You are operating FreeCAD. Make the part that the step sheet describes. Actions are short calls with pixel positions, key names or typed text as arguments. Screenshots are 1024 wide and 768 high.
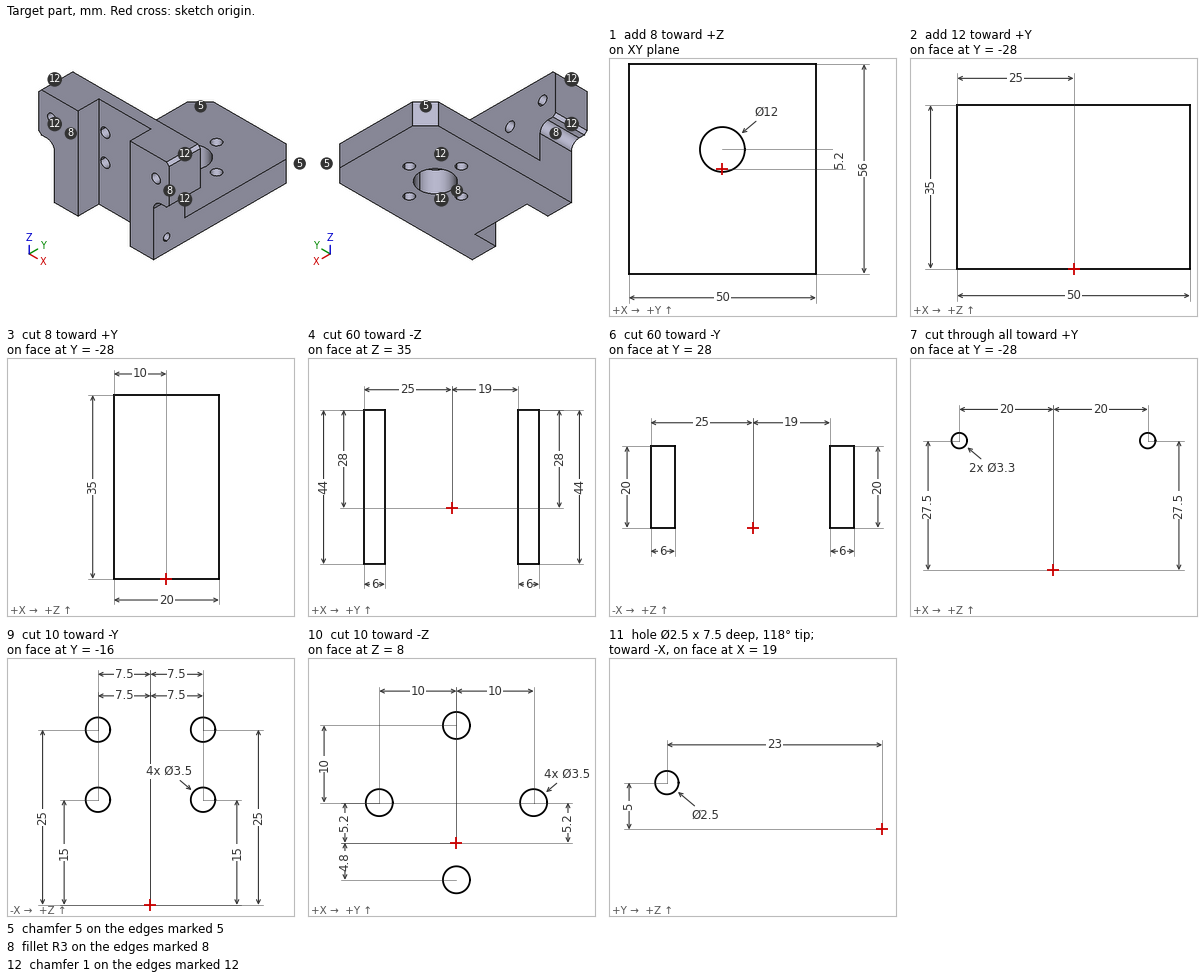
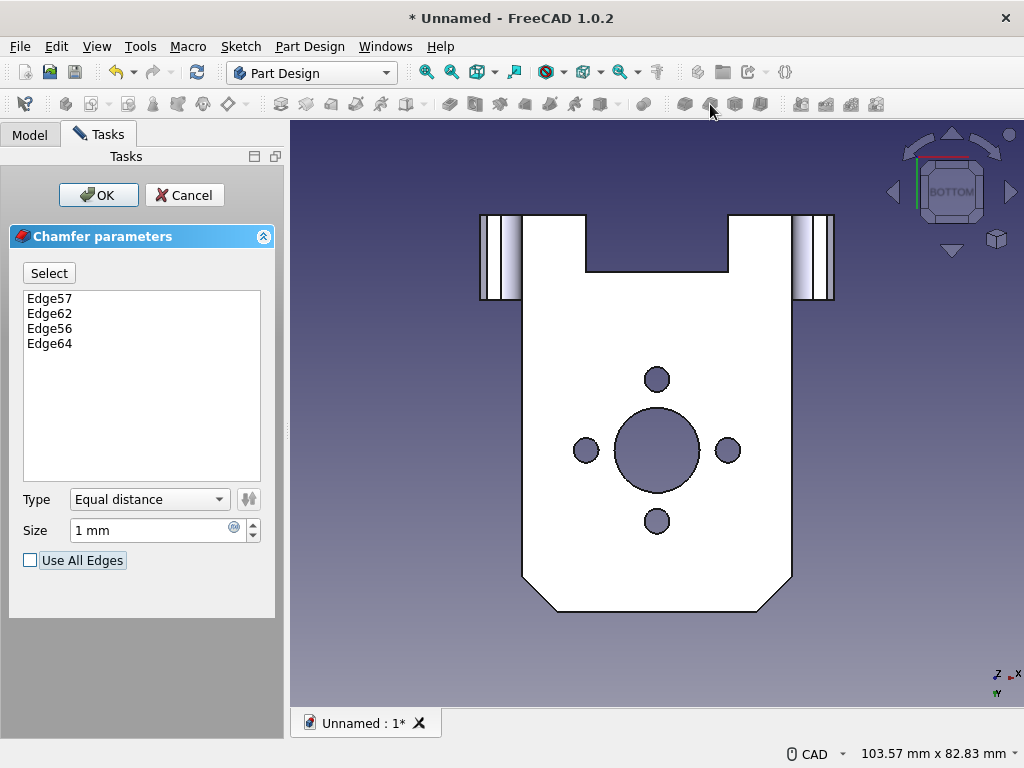
click(99, 195)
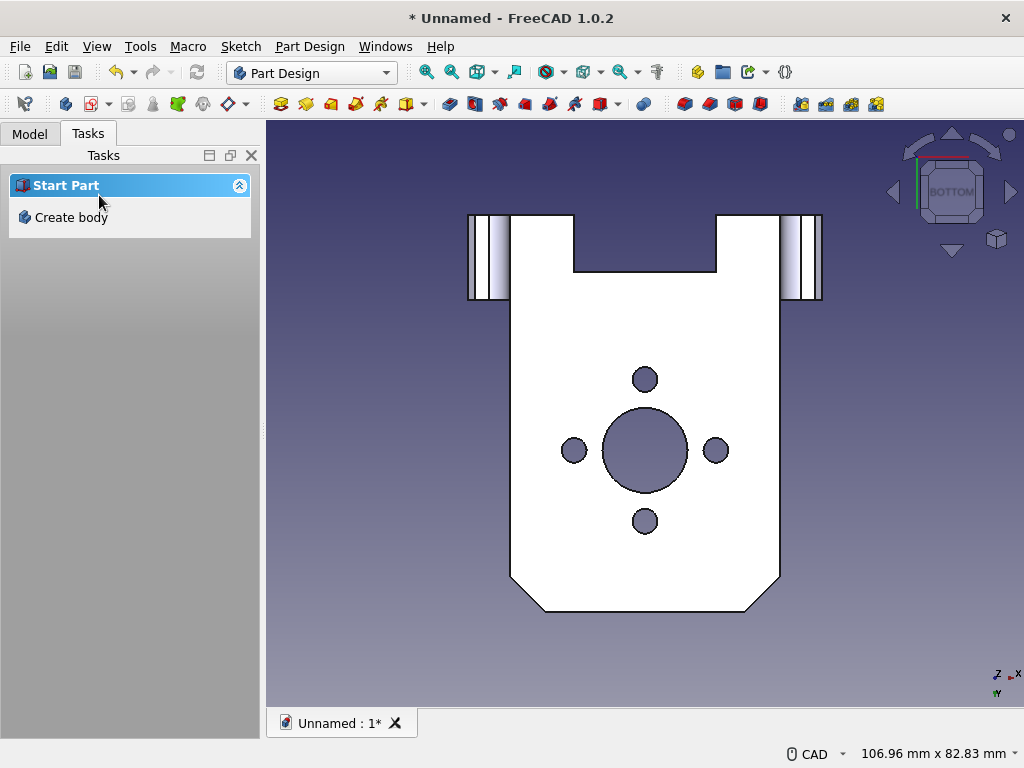
key(0)